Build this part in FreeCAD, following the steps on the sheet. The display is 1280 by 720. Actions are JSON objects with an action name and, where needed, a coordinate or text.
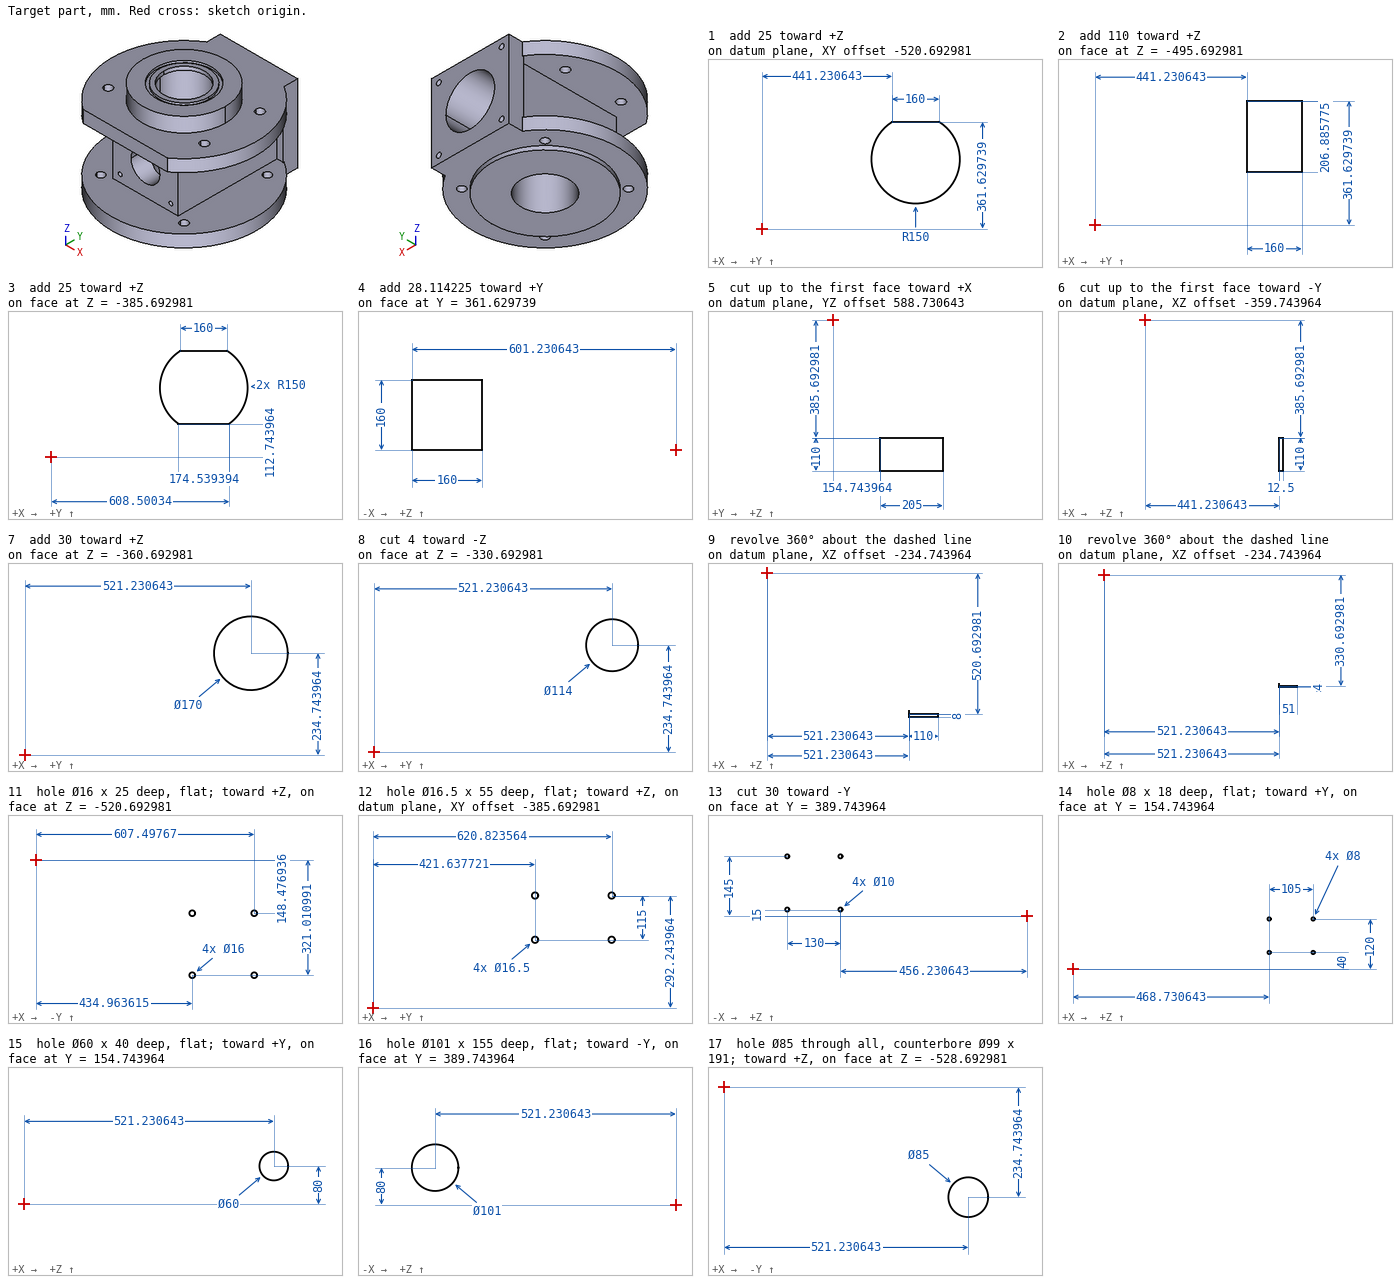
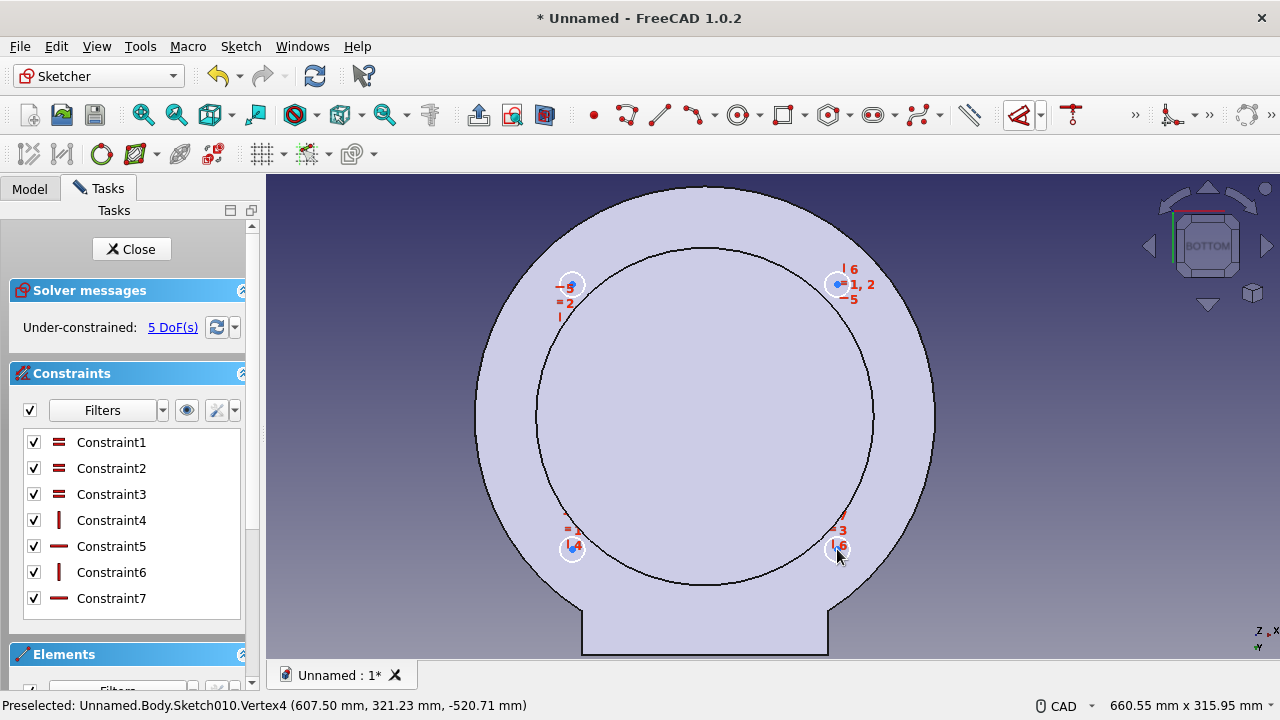
{"action": "scroll", "coordinate": [581, 541], "scroll_direction": "up", "scroll_amount": 3}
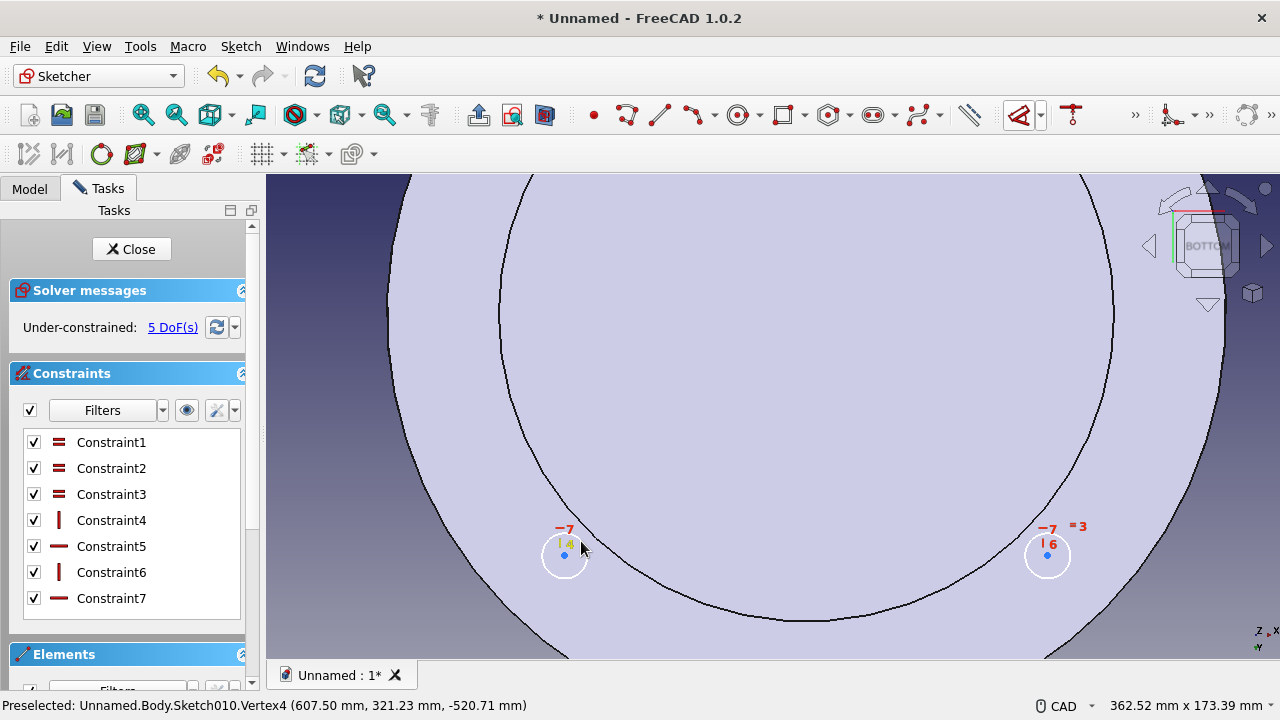
{"action": "left_click", "coordinate": [581, 540]}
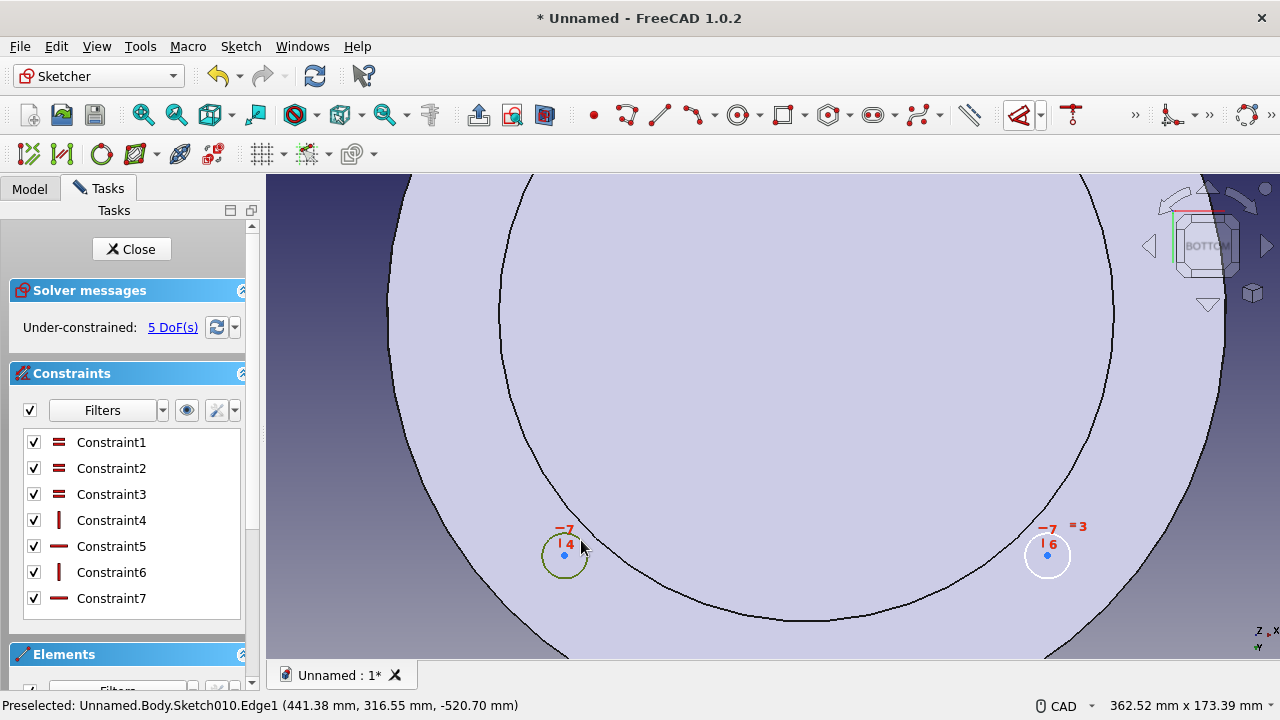
{"action": "left_click", "coordinate": [1040, 116]}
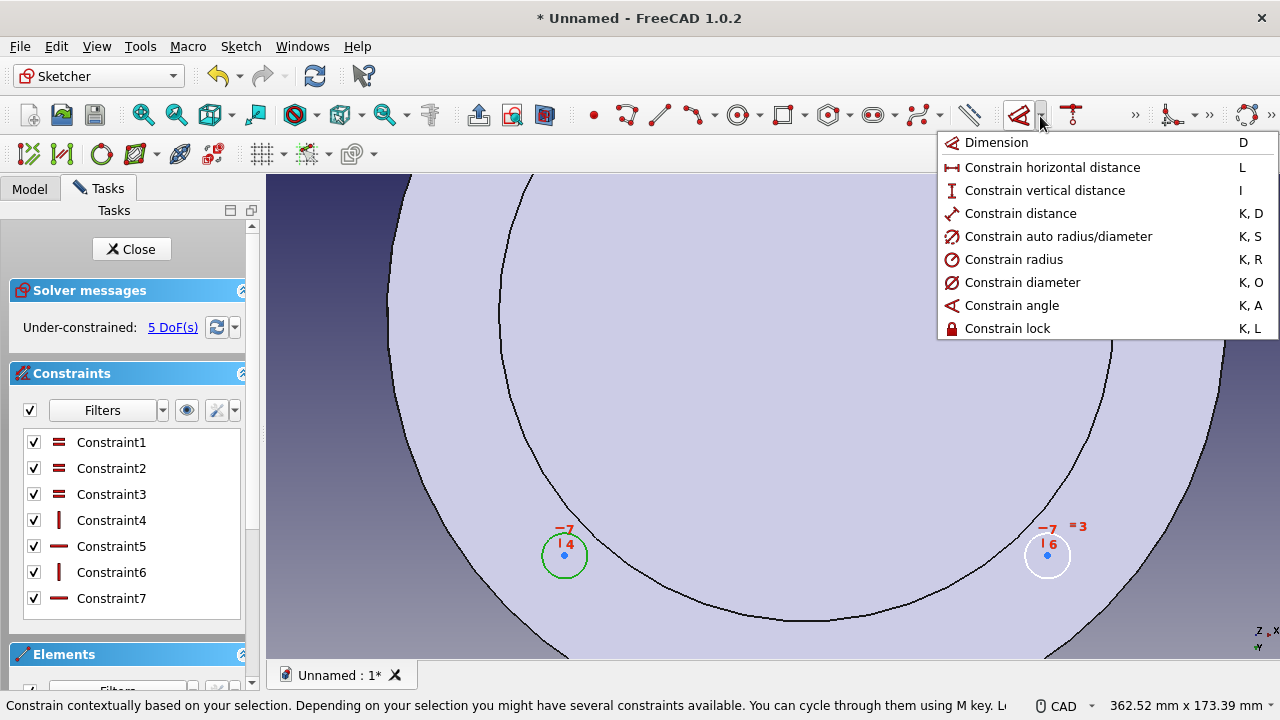
{"action": "left_click", "coordinate": [1108, 282]}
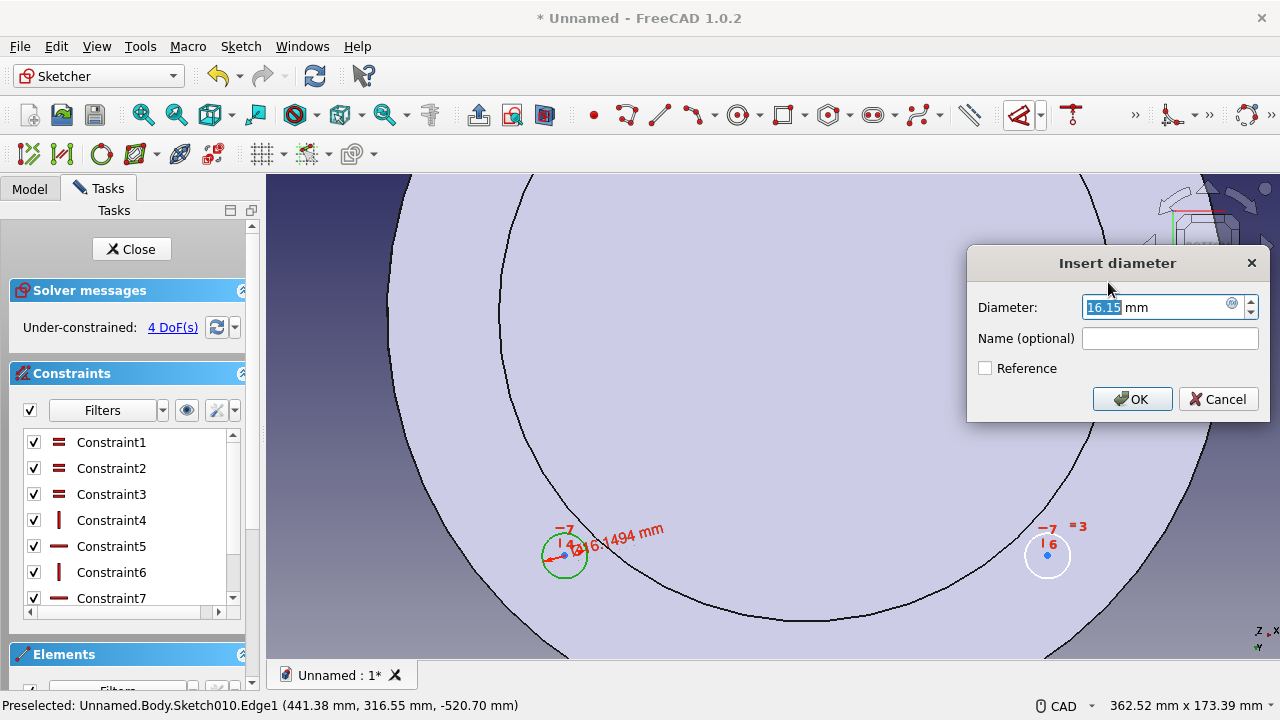
{"action": "type", "text": "16"}
{"action": "key", "text": "Return"}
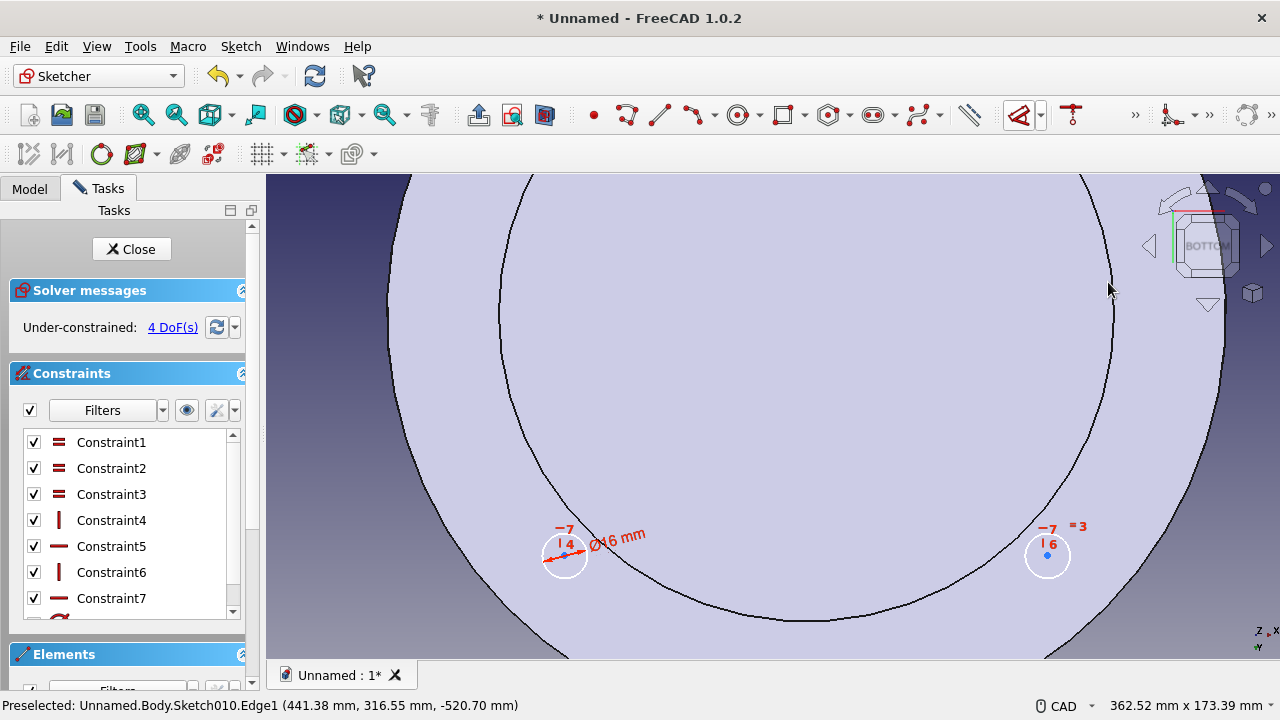
{"action": "scroll", "coordinate": [580, 541], "scroll_direction": "down", "scroll_amount": 3}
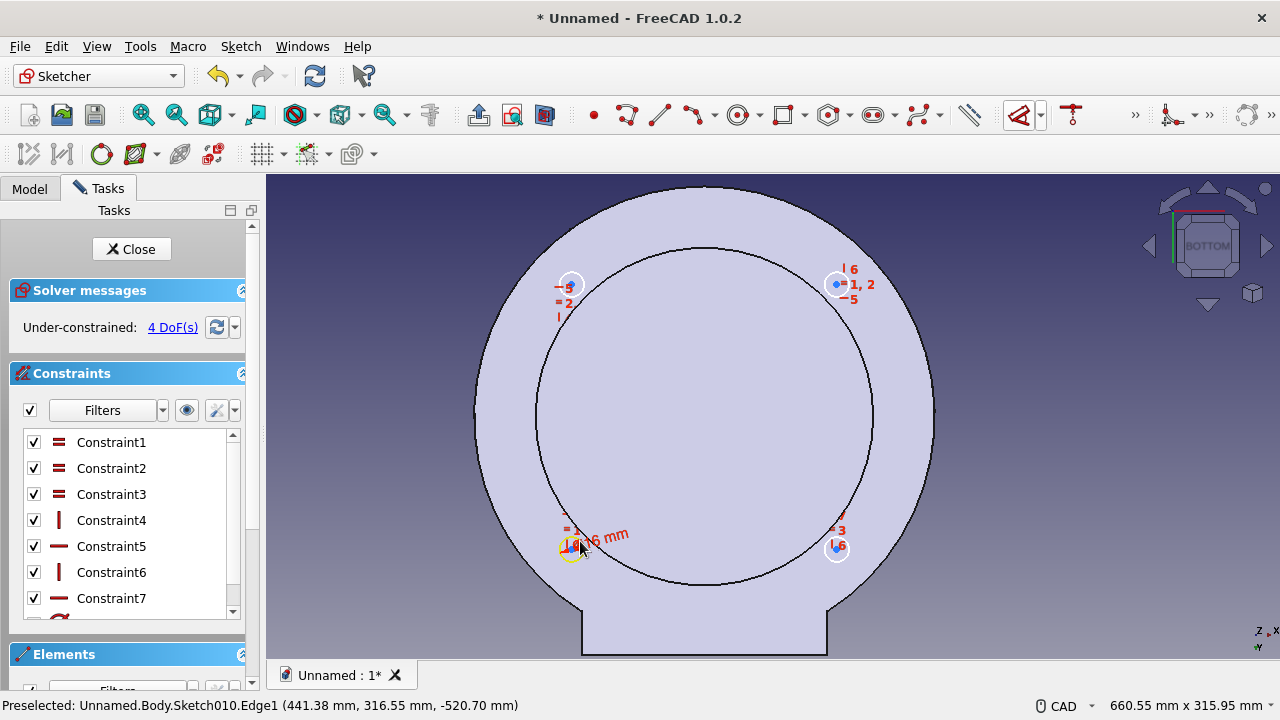
{"action": "left_click", "coordinate": [837, 285]}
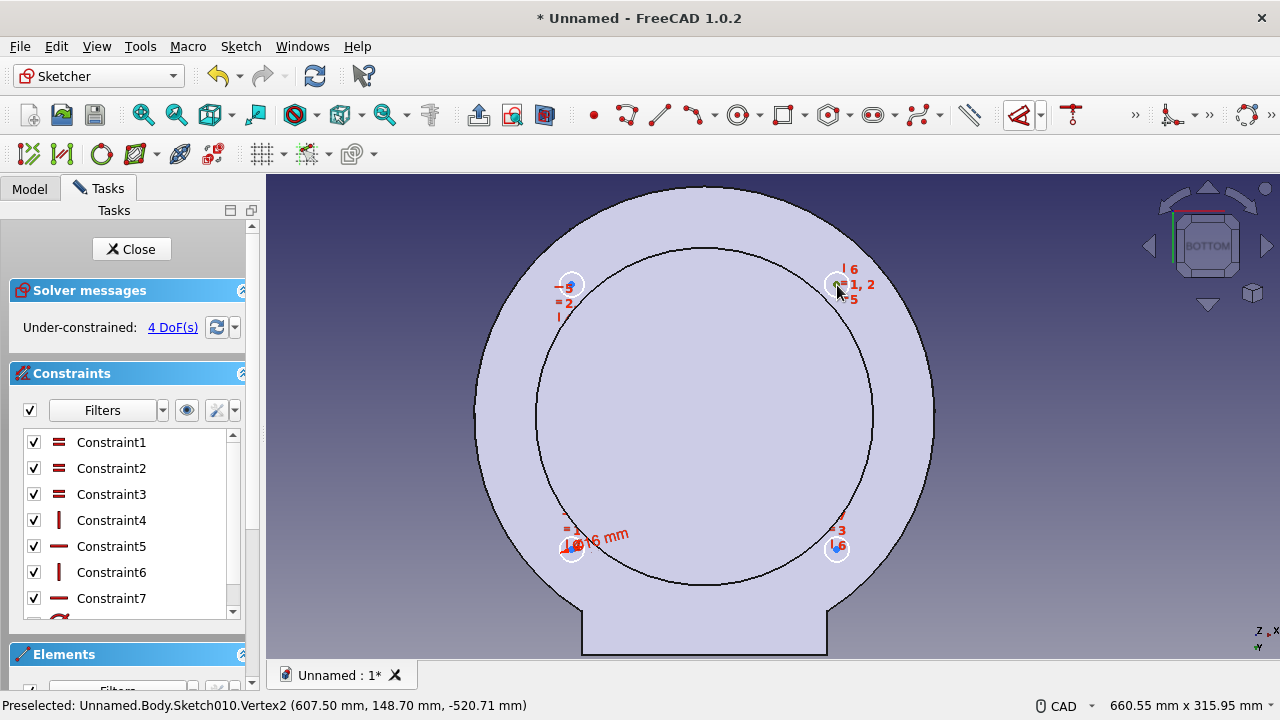
{"action": "left_click", "coordinate": [1040, 116]}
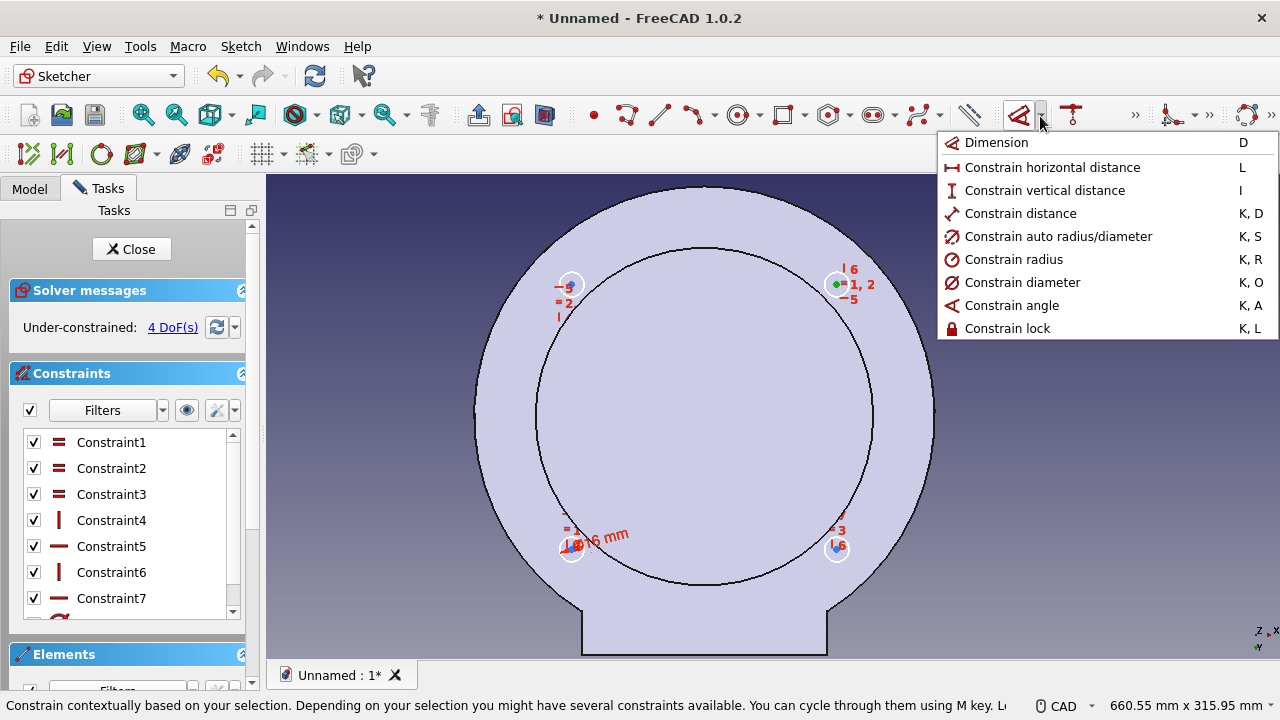
{"action": "left_click", "coordinate": [1108, 168]}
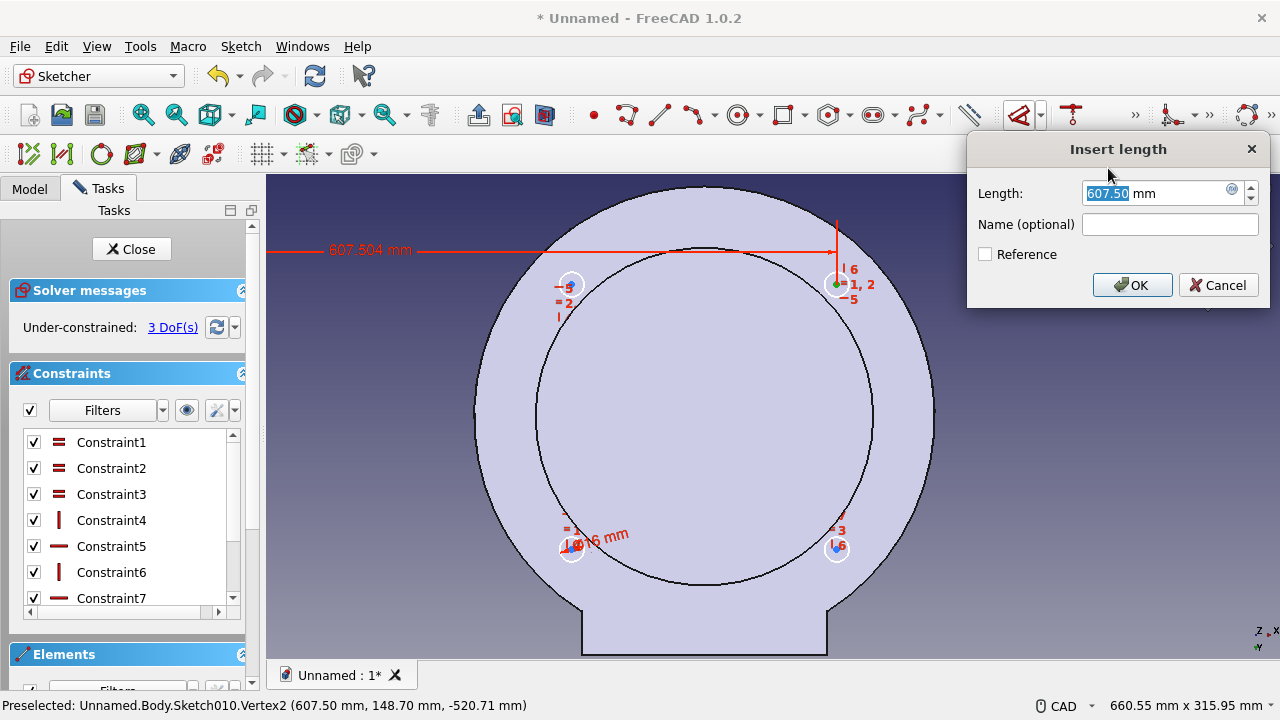
{"action": "type", "text": "607.49767"}
{"action": "key", "text": "Return"}